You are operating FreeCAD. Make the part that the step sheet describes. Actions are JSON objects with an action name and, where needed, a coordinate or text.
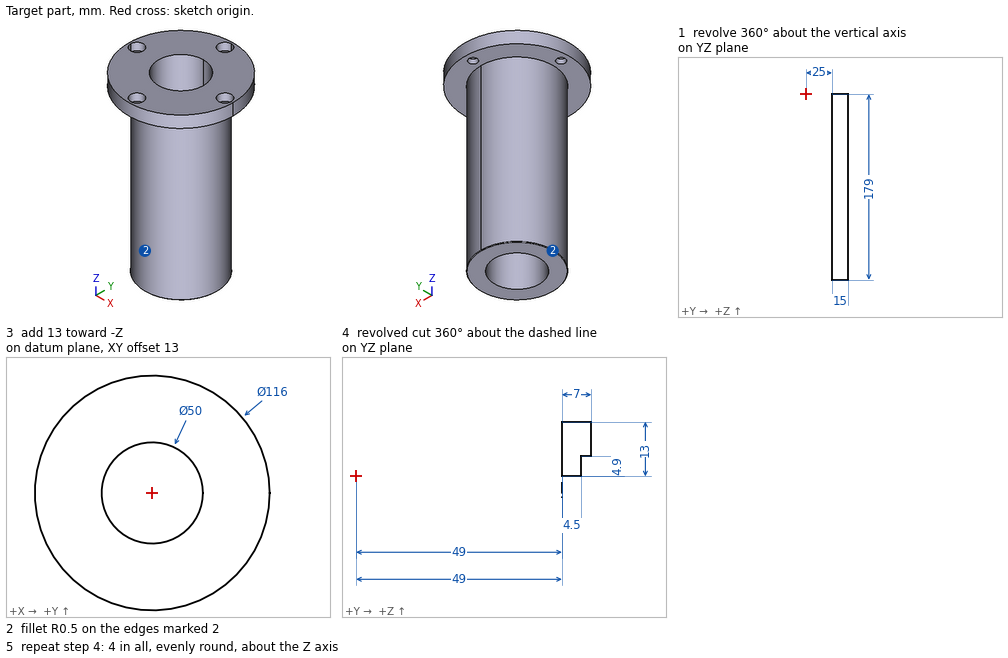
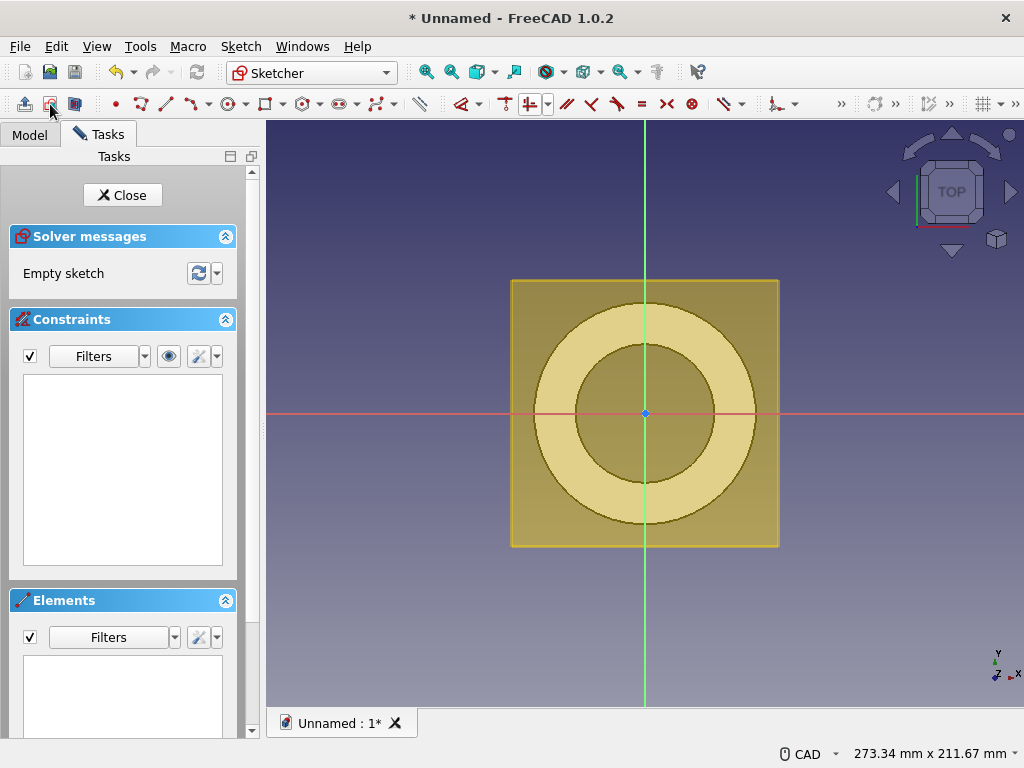
{"action": "left_click", "coordinate": [228, 104]}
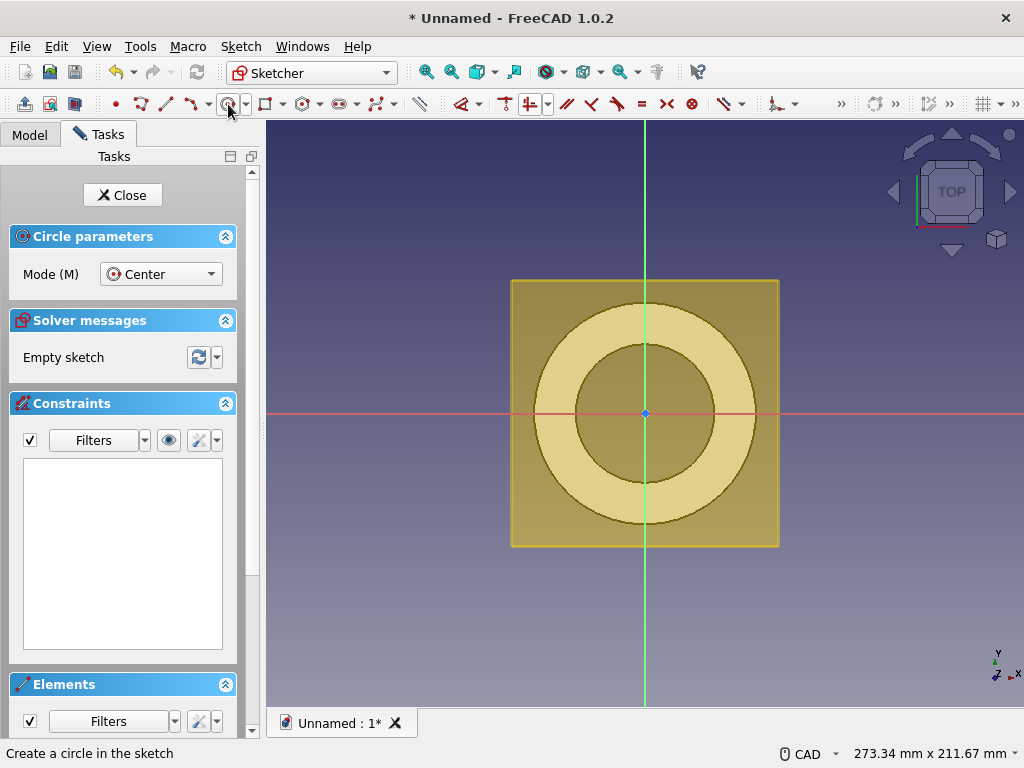
{"action": "left_click", "coordinate": [645, 413]}
{"action": "left_click", "coordinate": [759, 300]}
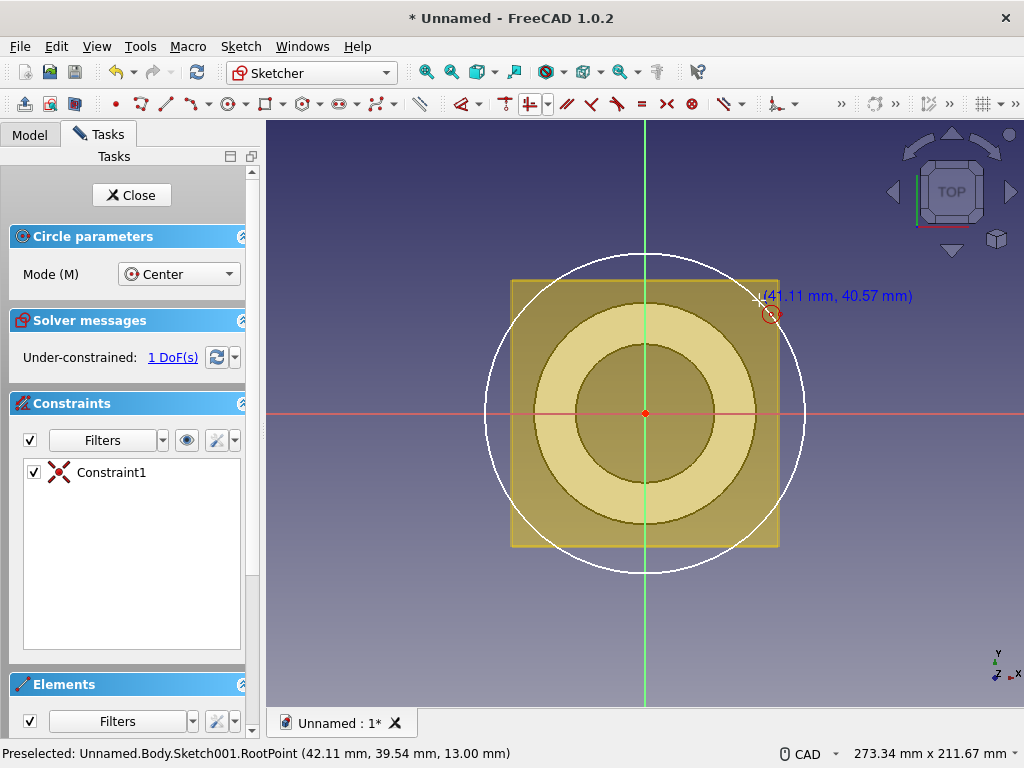
{"action": "left_click", "coordinate": [645, 413]}
{"action": "left_click", "coordinate": [694, 364]}
{"action": "key", "text": "Escape"}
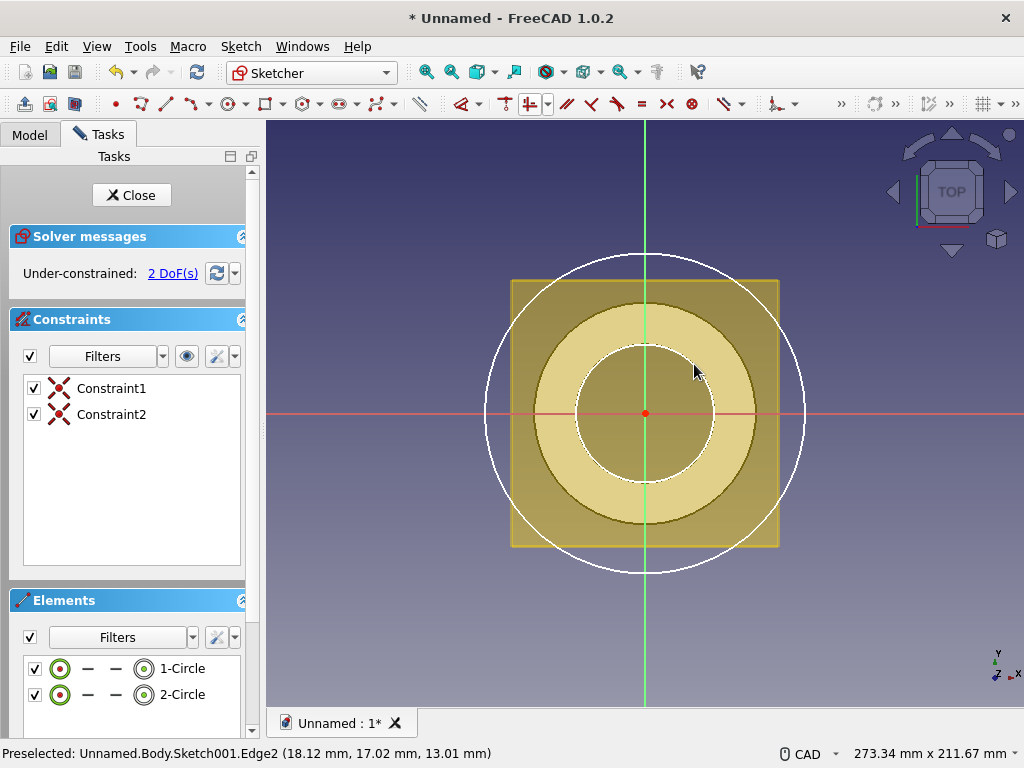
{"action": "left_click", "coordinate": [460, 104]}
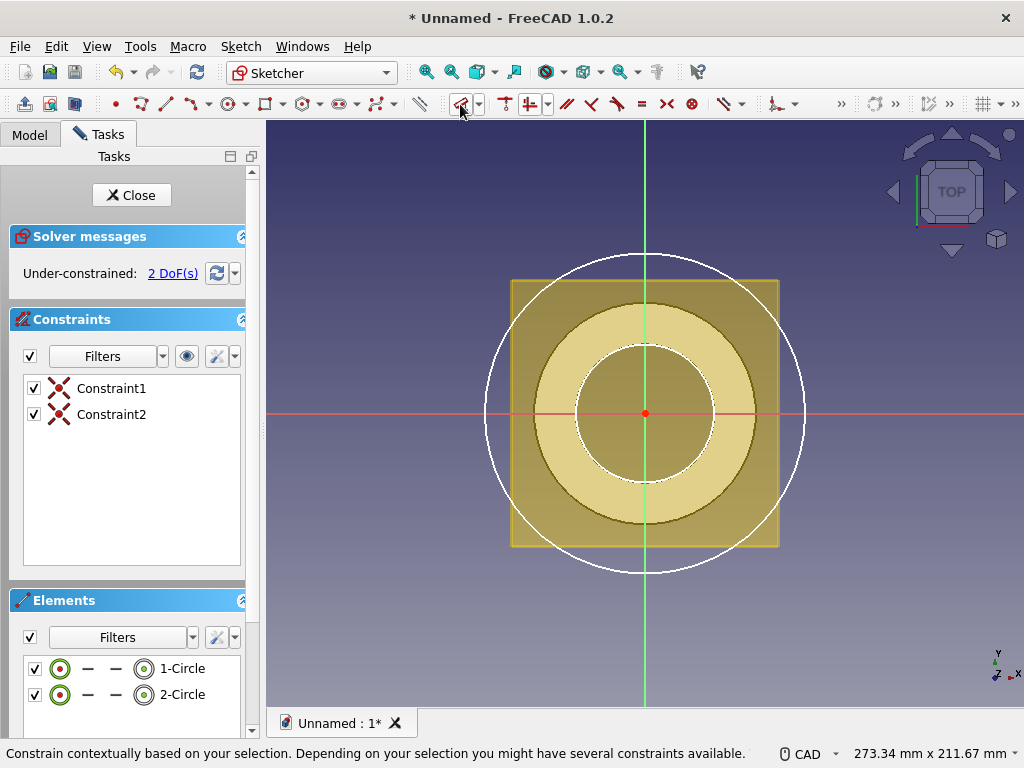
{"action": "left_click", "coordinate": [758, 300]}
{"action": "left_click", "coordinate": [781, 277]}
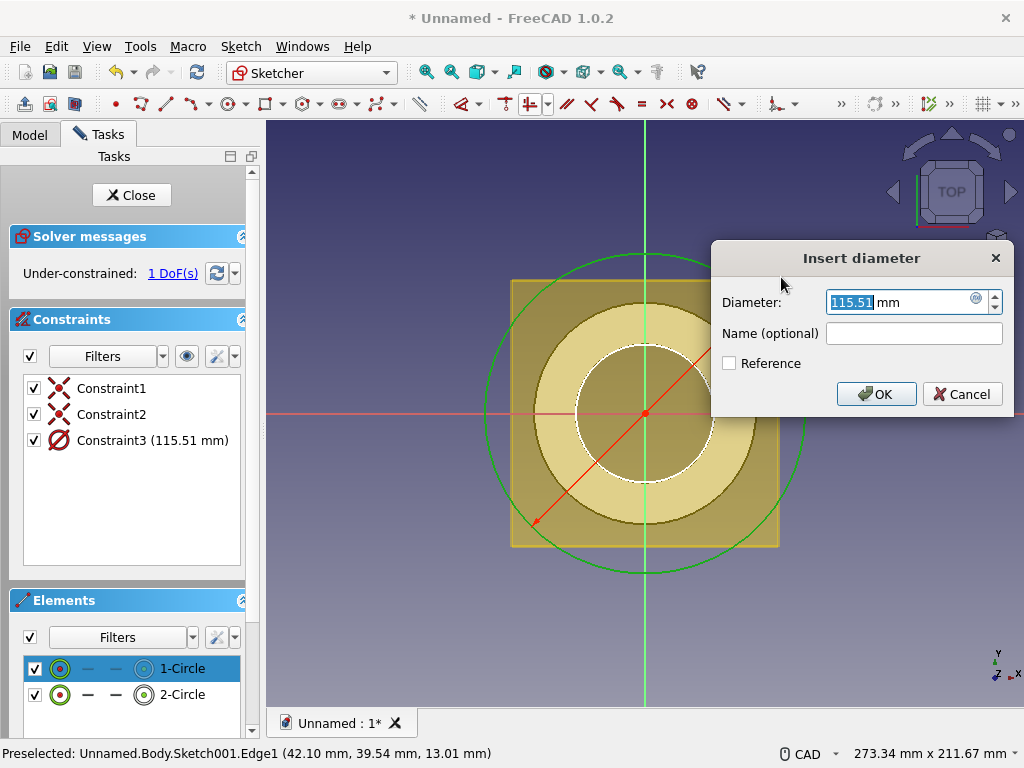
{"action": "type", "text": "116"}
{"action": "key", "text": "Return"}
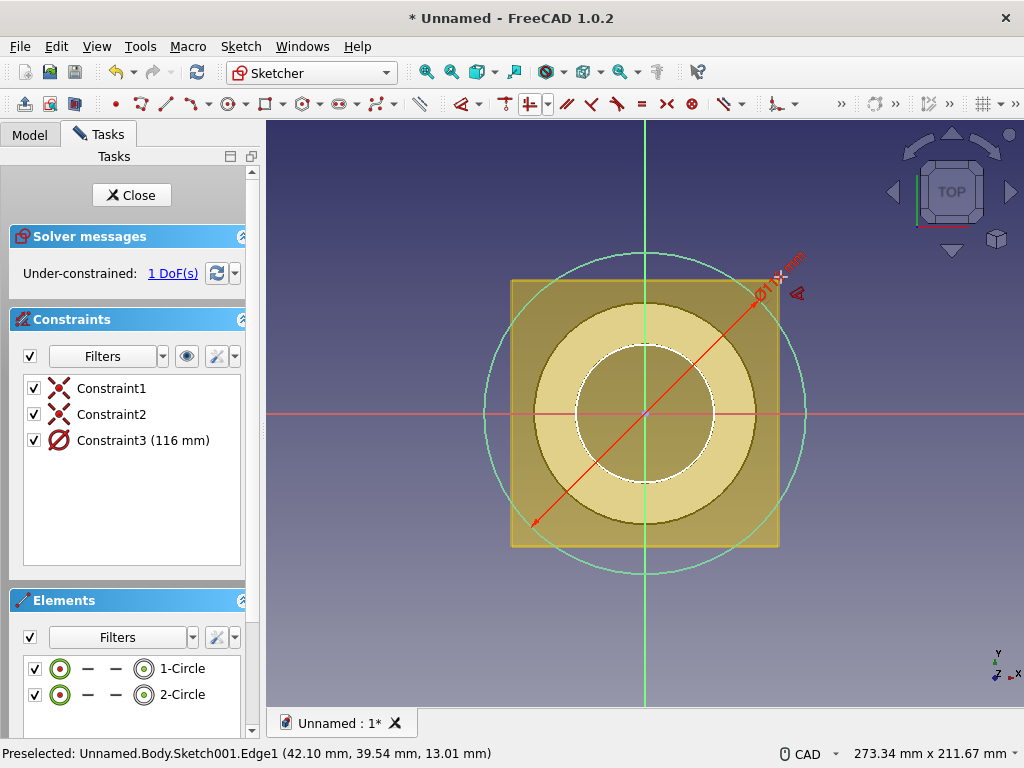
{"action": "left_click", "coordinate": [694, 365]}
{"action": "left_click", "coordinate": [717, 342]}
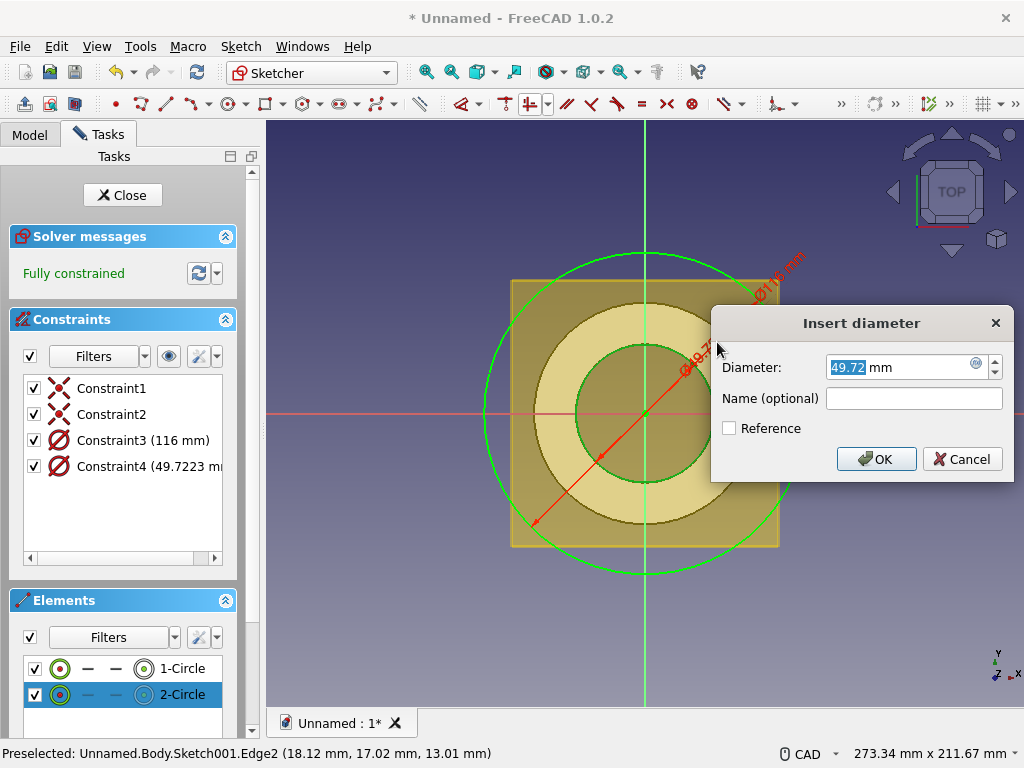
{"action": "type", "text": "50"}
{"action": "key", "text": "Return"}
{"action": "key", "text": "Escape"}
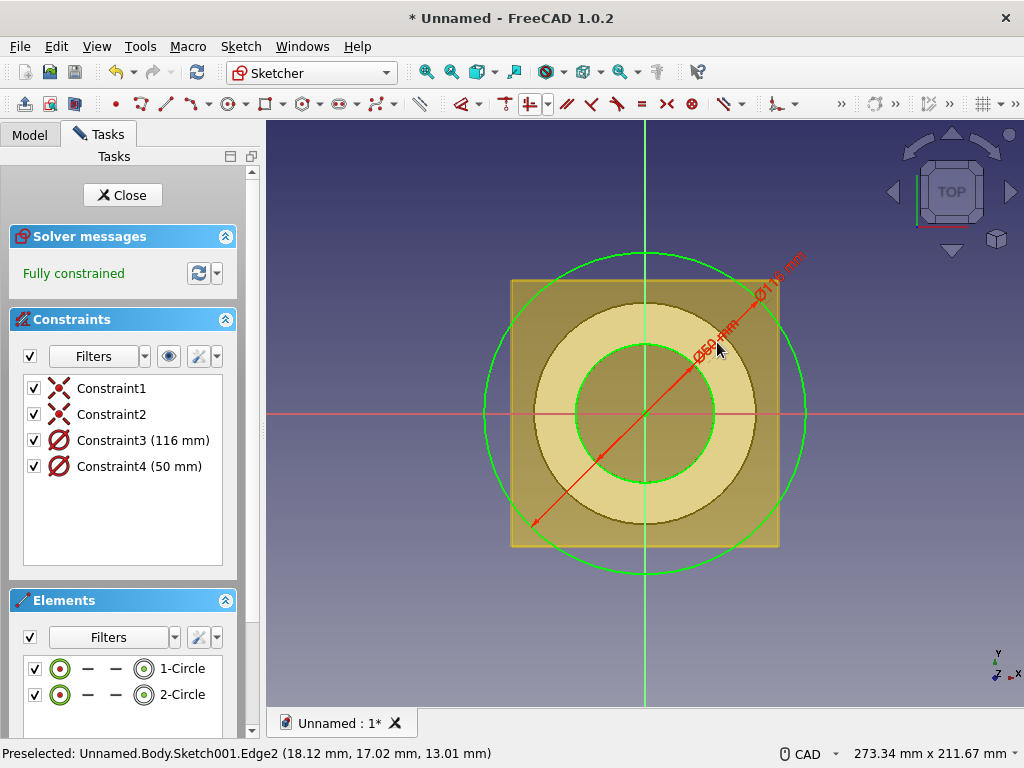
{"action": "left_click", "coordinate": [123, 195]}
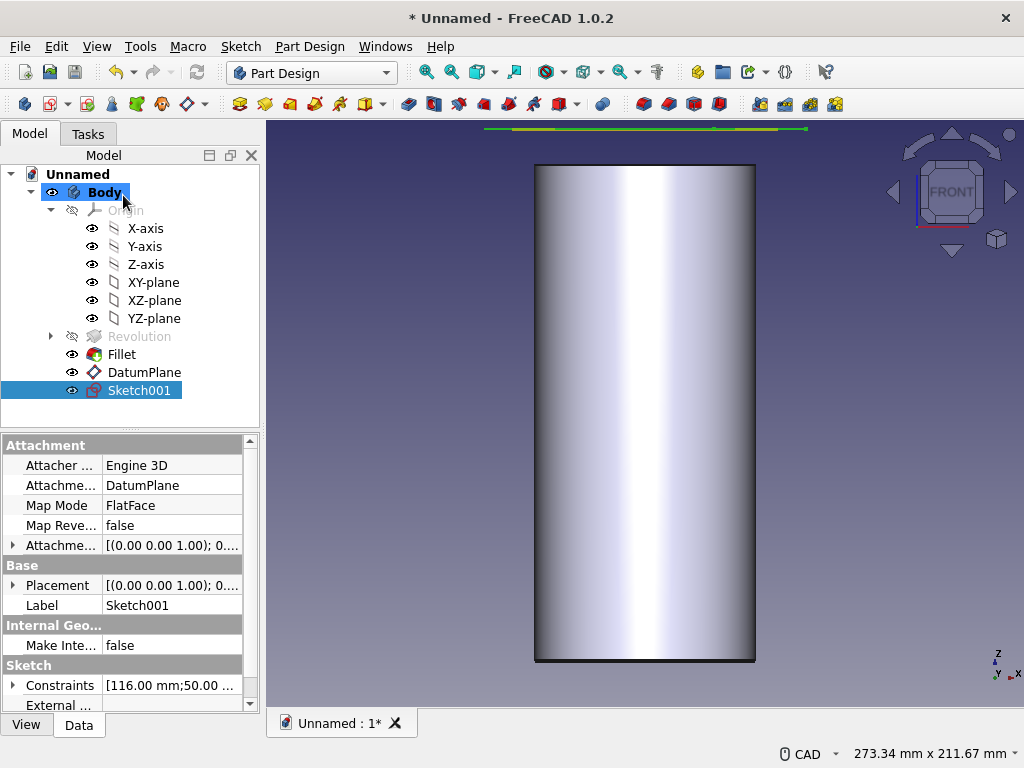
{"action": "left_click", "coordinate": [240, 104]}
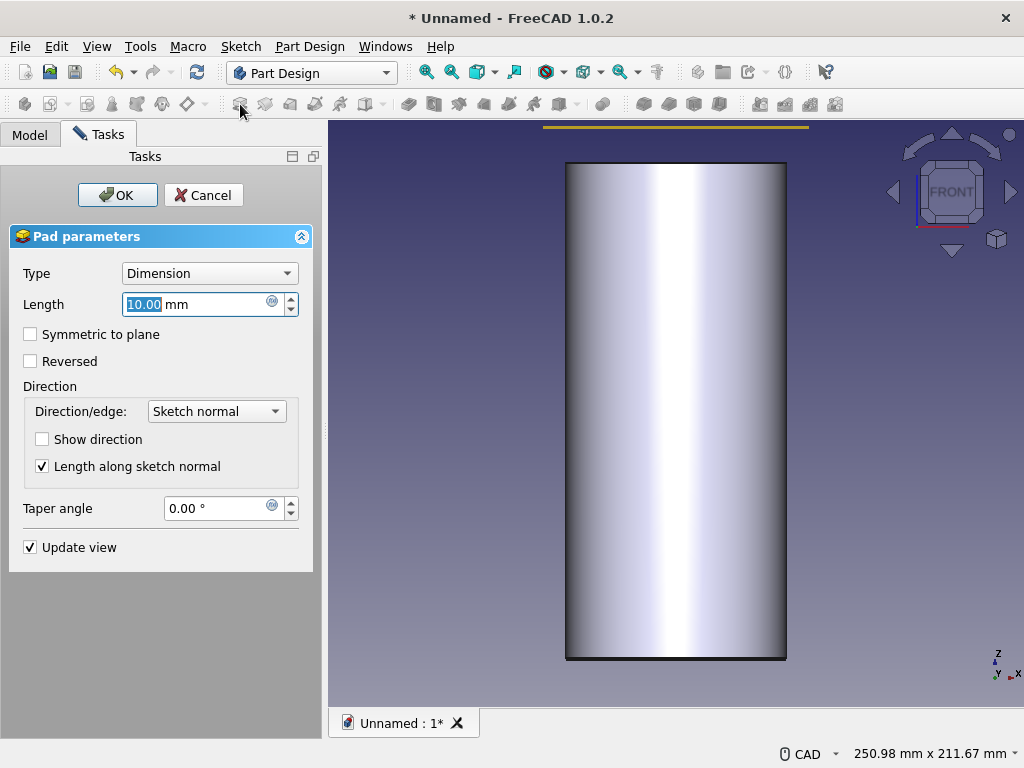
{"action": "type", "text": "13"}
{"action": "key", "text": "Tab"}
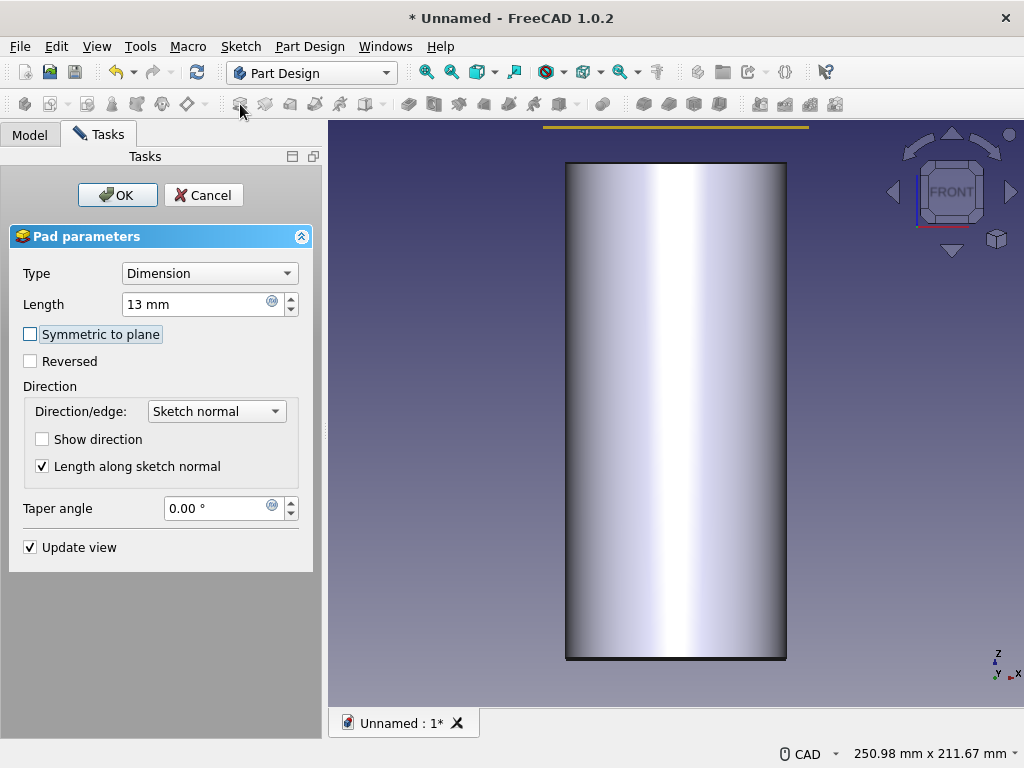
{"action": "left_click", "coordinate": [31, 361]}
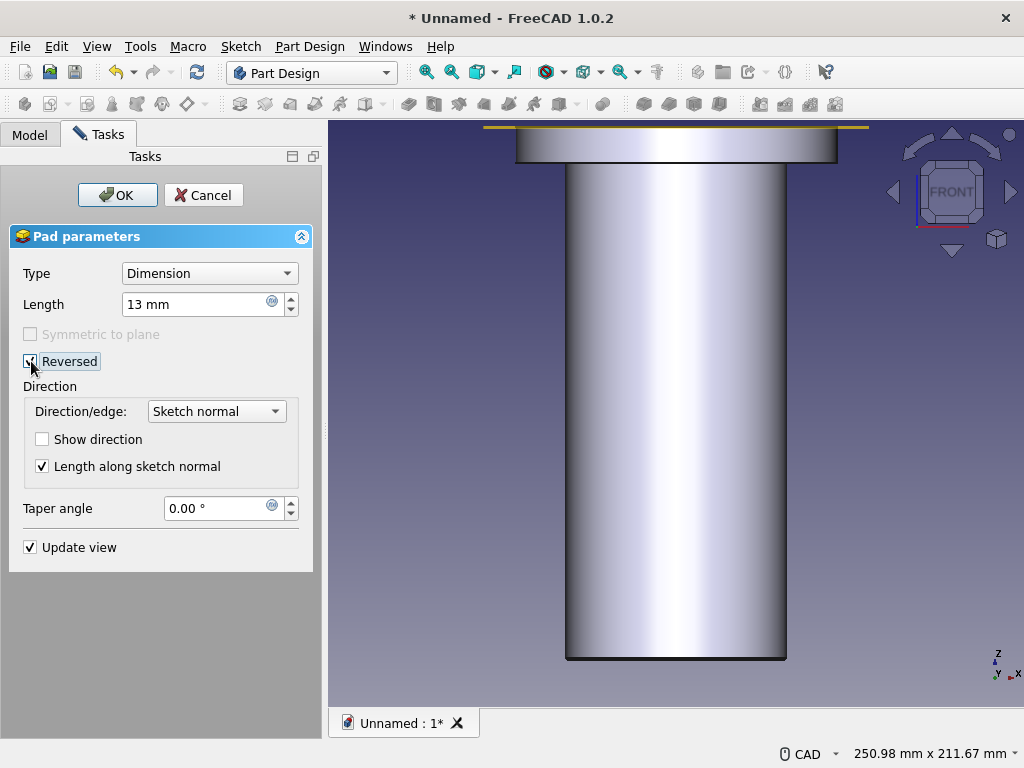
{"action": "left_click", "coordinate": [118, 195]}